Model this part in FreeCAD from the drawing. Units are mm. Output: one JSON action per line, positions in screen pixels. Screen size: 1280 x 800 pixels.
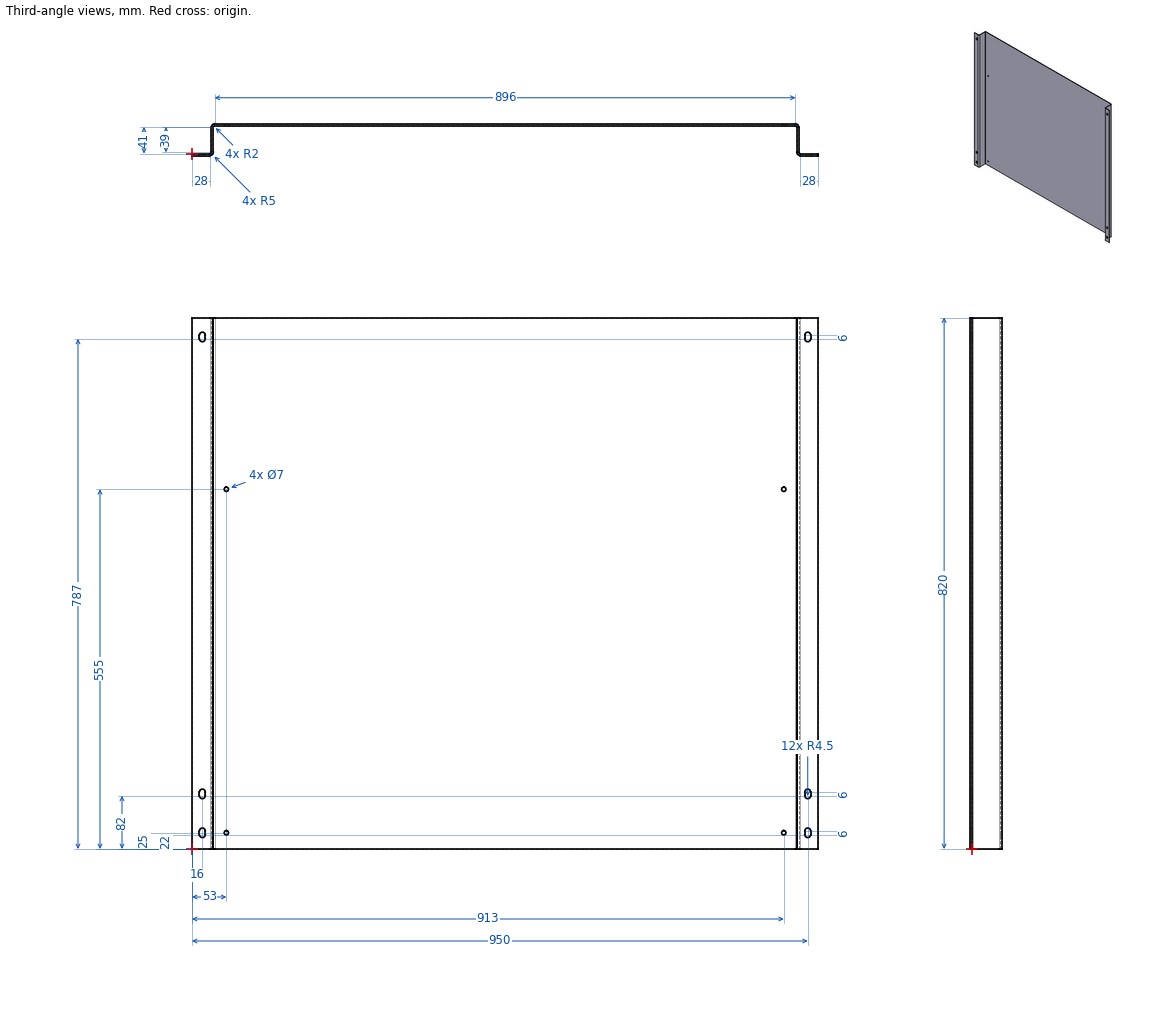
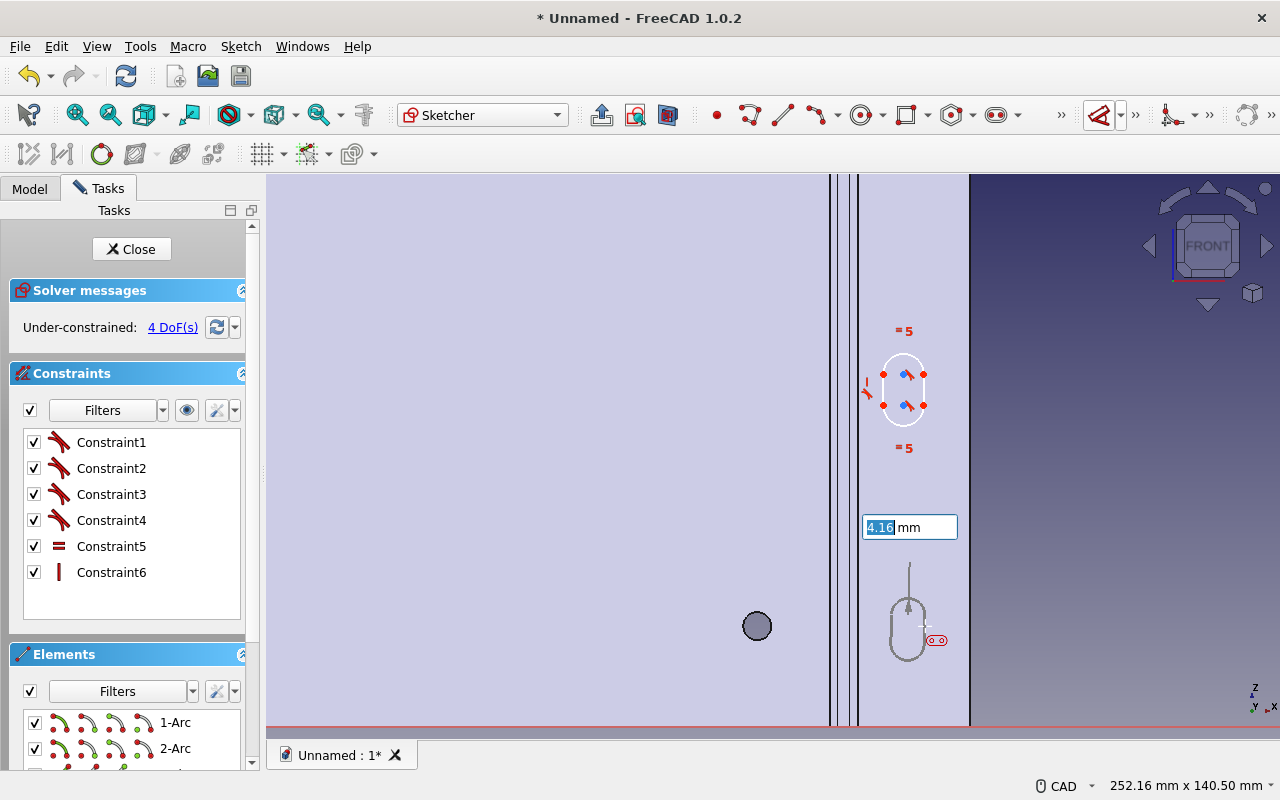
{"action": "left_click", "coordinate": [924, 626]}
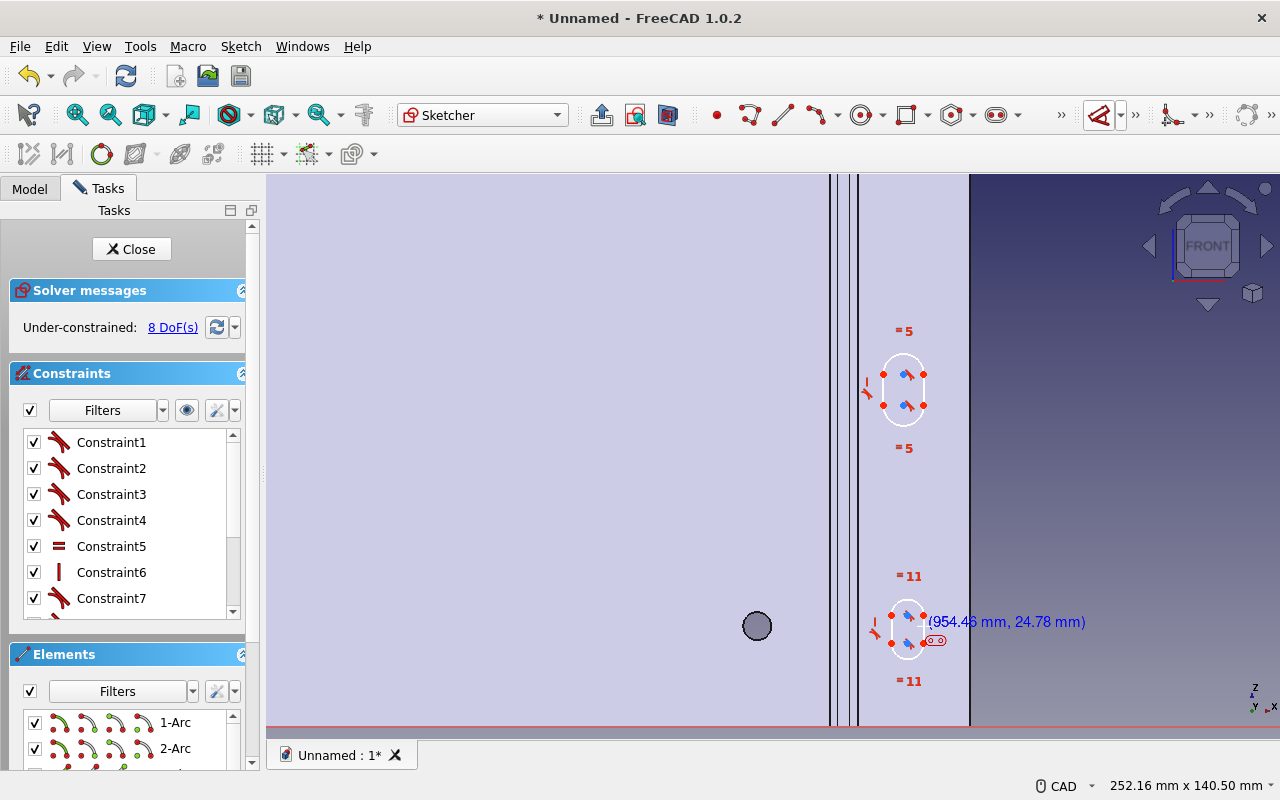
{"action": "scroll", "coordinate": [916, 623], "scroll_direction": "down", "scroll_amount": 11}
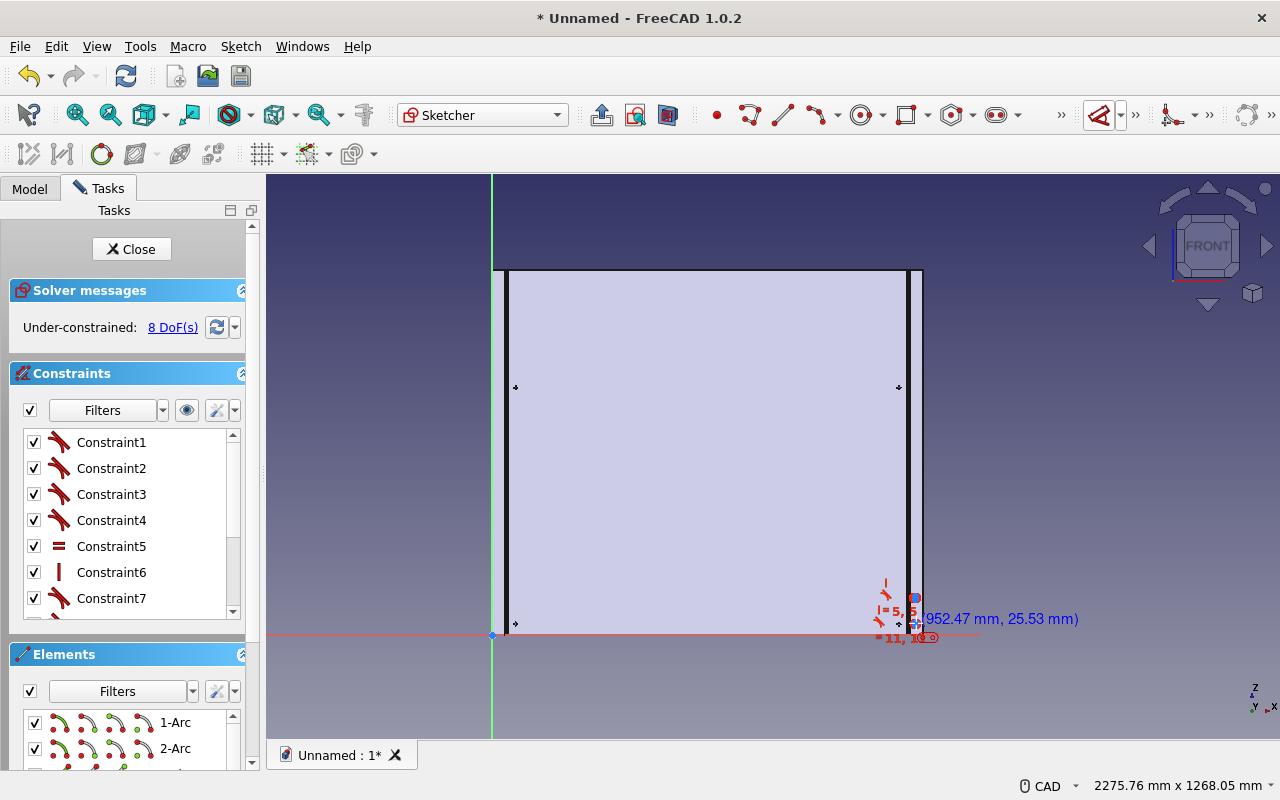
{"action": "scroll", "coordinate": [499, 599], "scroll_direction": "up", "scroll_amount": 13}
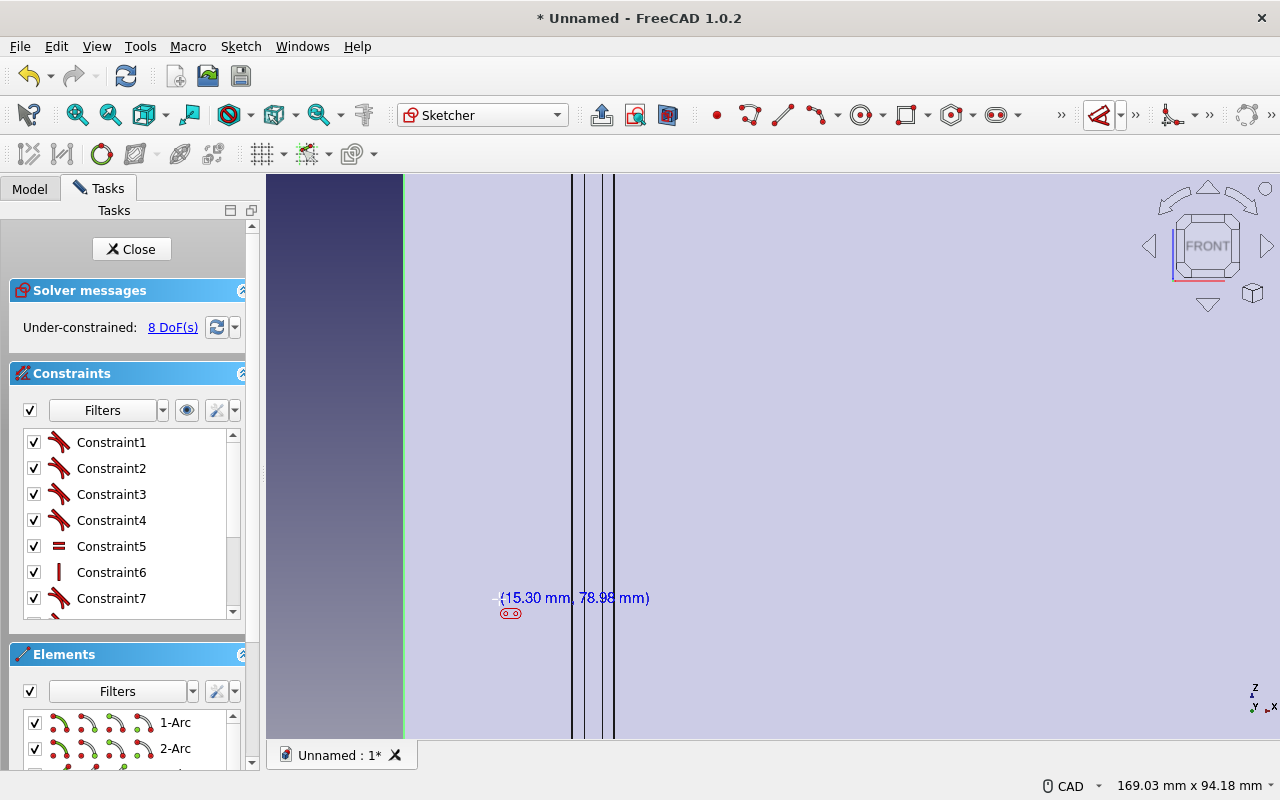
{"action": "scroll", "coordinate": [499, 599], "scroll_direction": "down", "scroll_amount": 13}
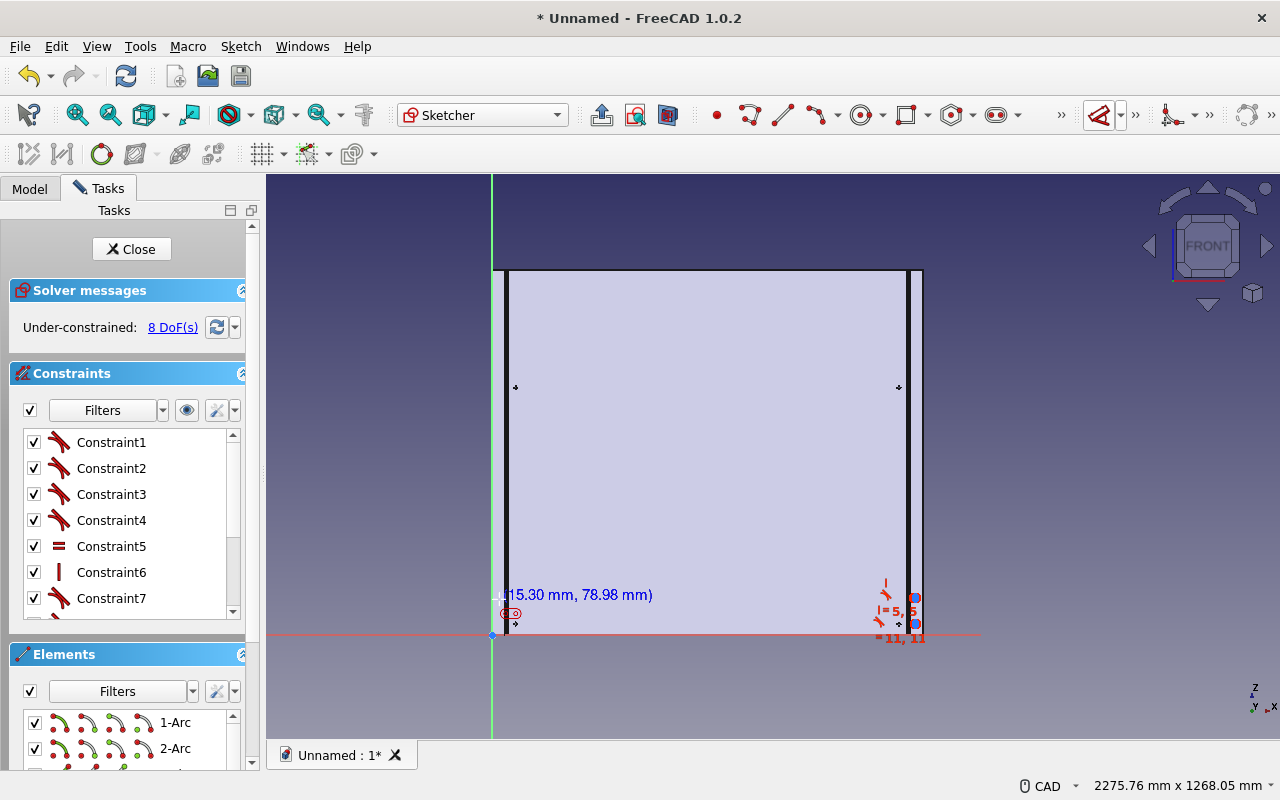
{"action": "scroll", "coordinate": [499, 599], "scroll_direction": "up", "scroll_amount": 5}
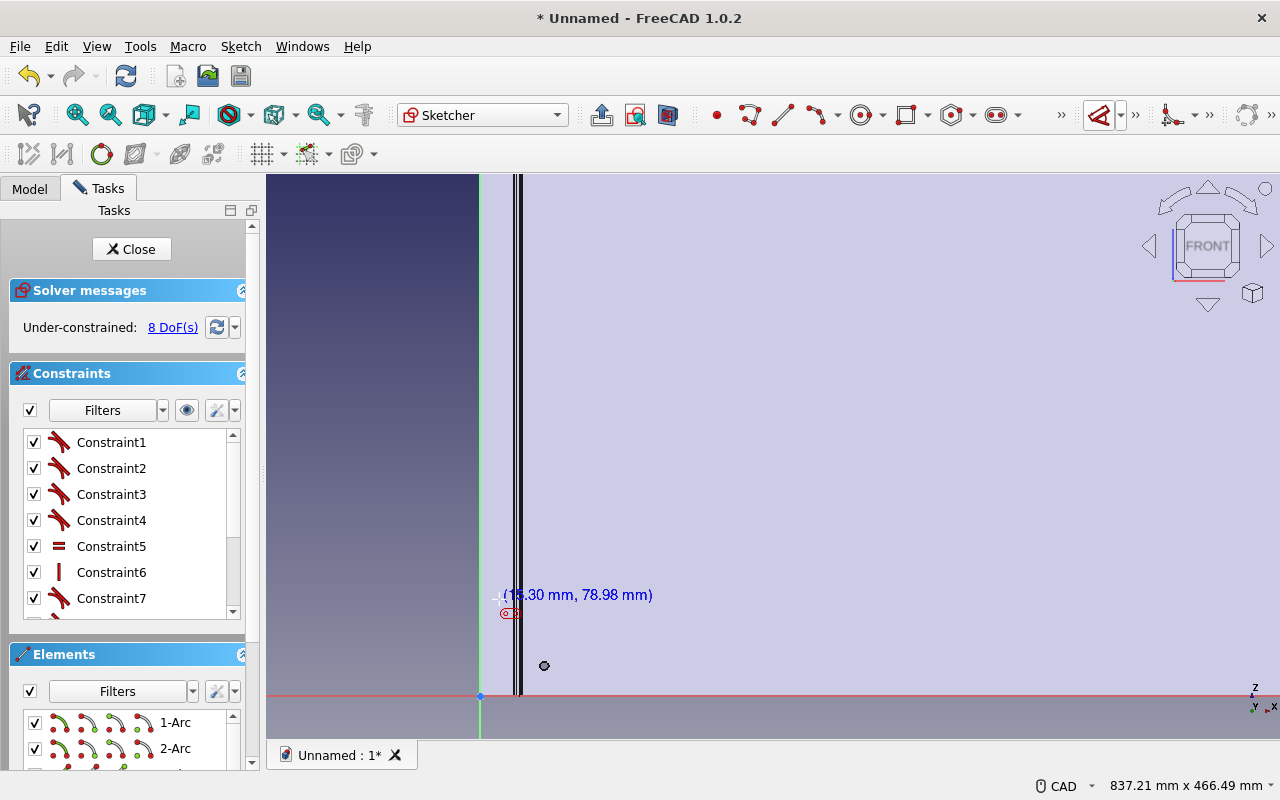
{"action": "left_click", "coordinate": [499, 597]}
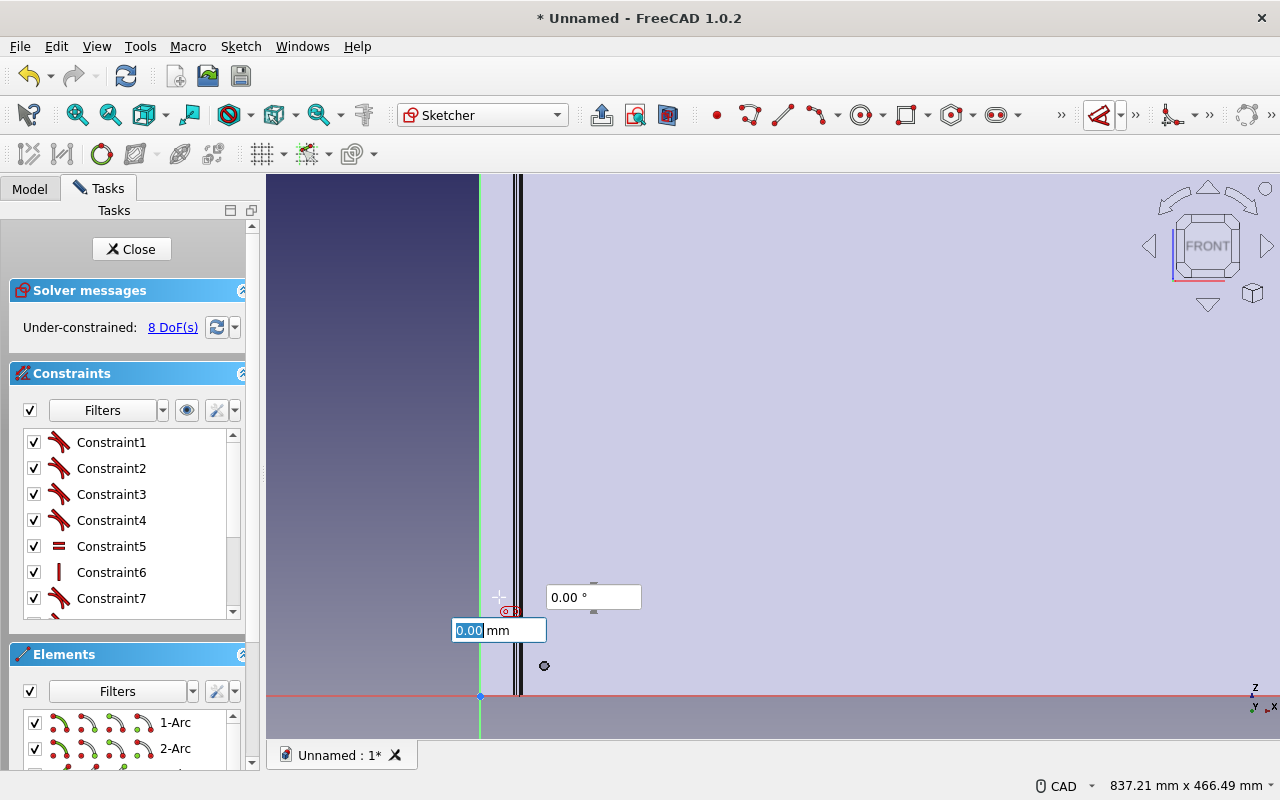
{"action": "scroll", "coordinate": [499, 590], "scroll_direction": "up", "scroll_amount": 4}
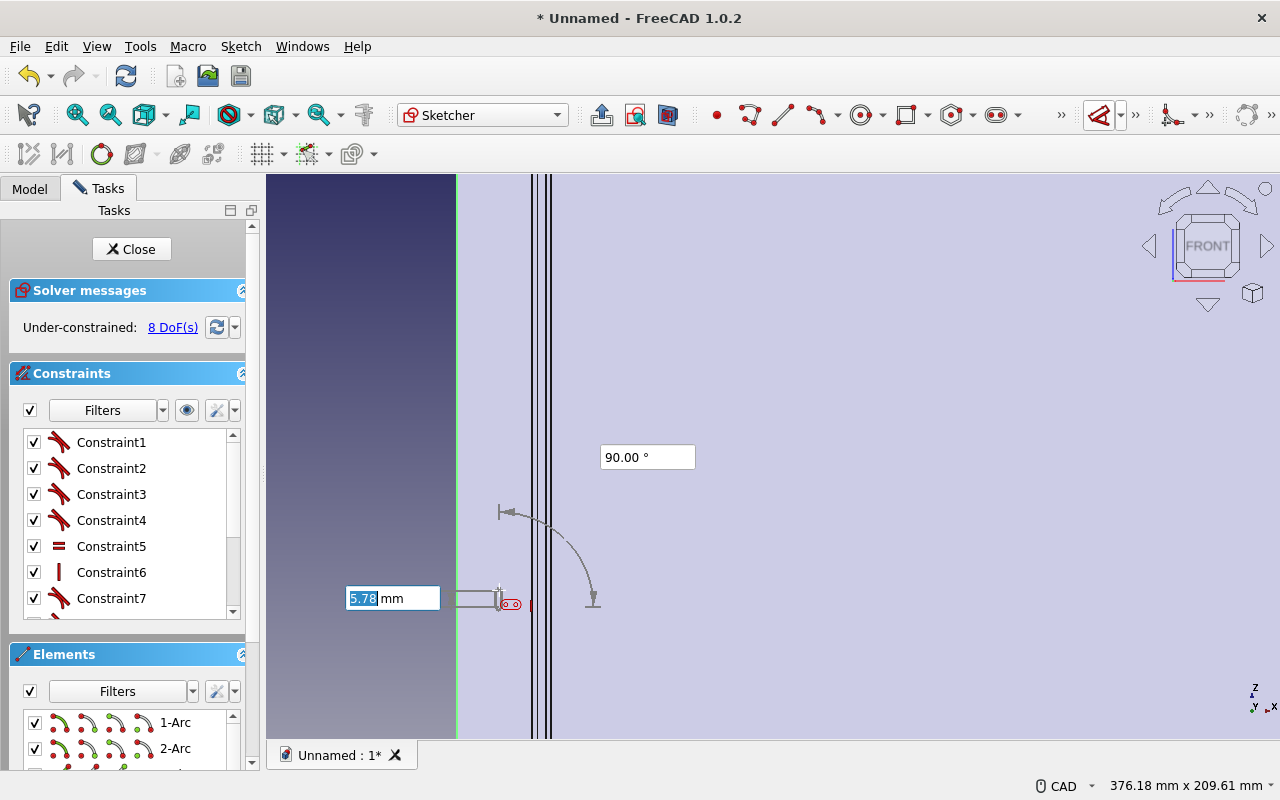
{"action": "left_click", "coordinate": [499, 588]}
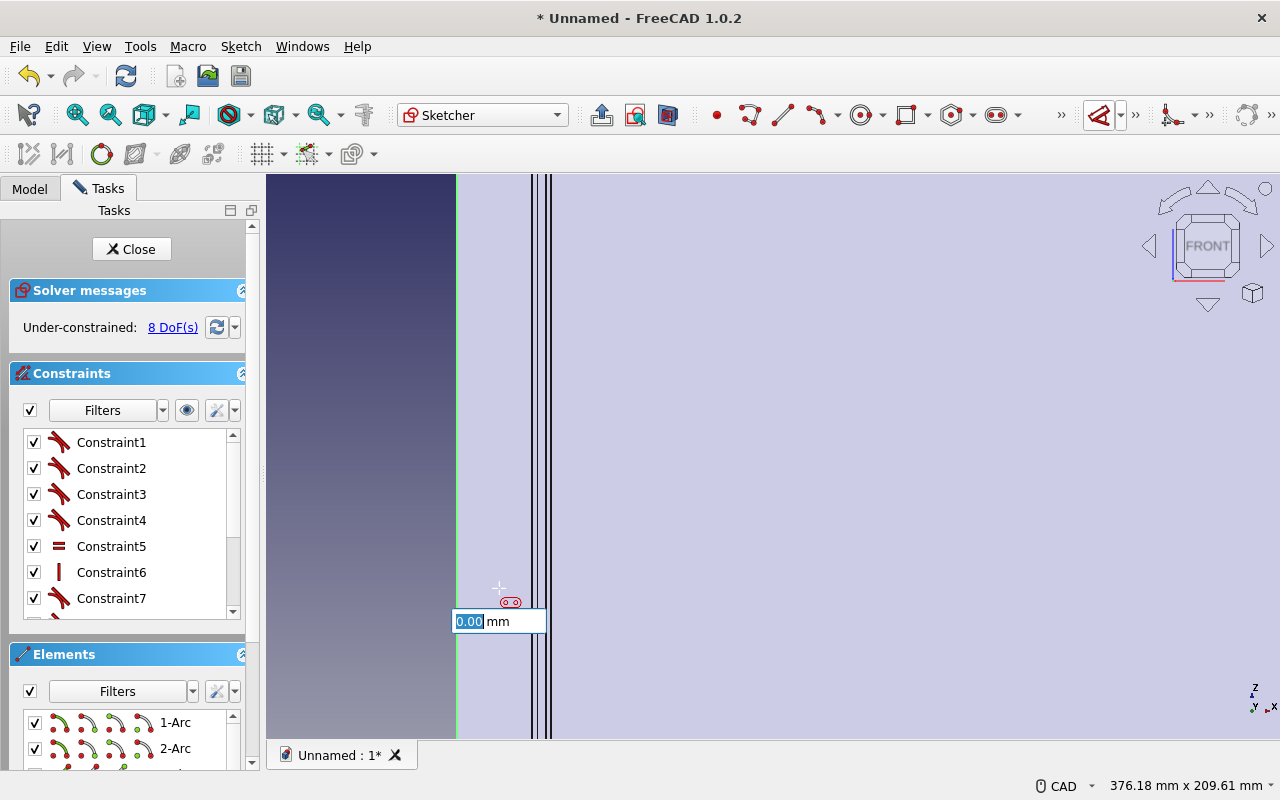
{"action": "scroll", "coordinate": [488, 596], "scroll_direction": "up", "scroll_amount": 2}